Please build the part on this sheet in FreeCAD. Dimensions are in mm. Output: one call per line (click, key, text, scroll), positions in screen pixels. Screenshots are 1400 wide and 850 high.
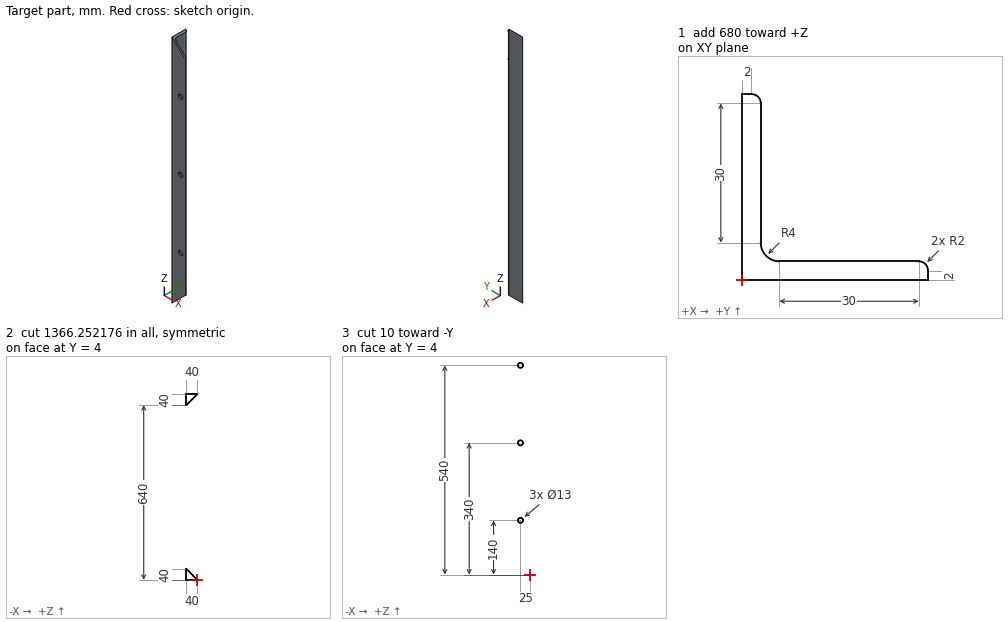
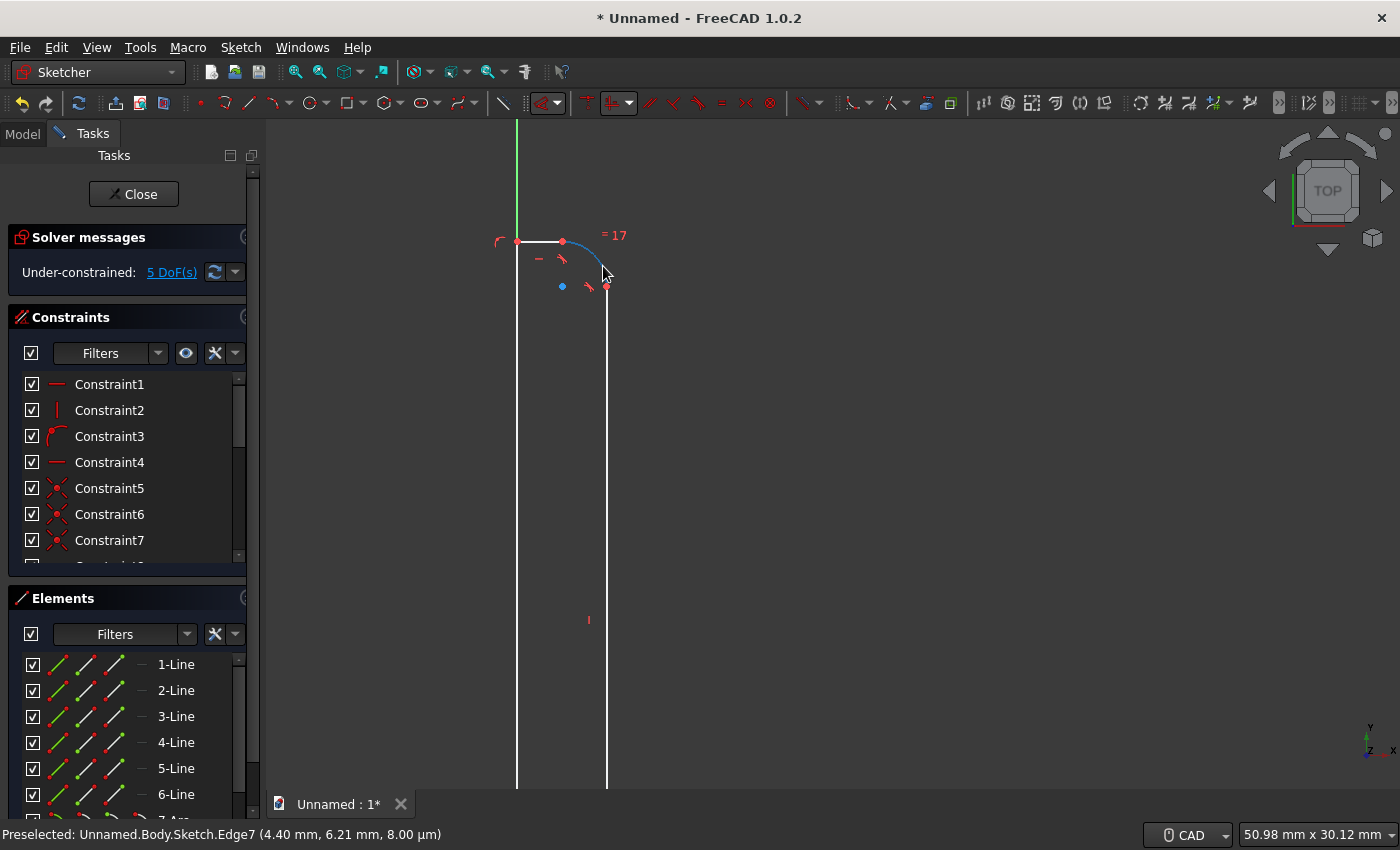
click(602, 266)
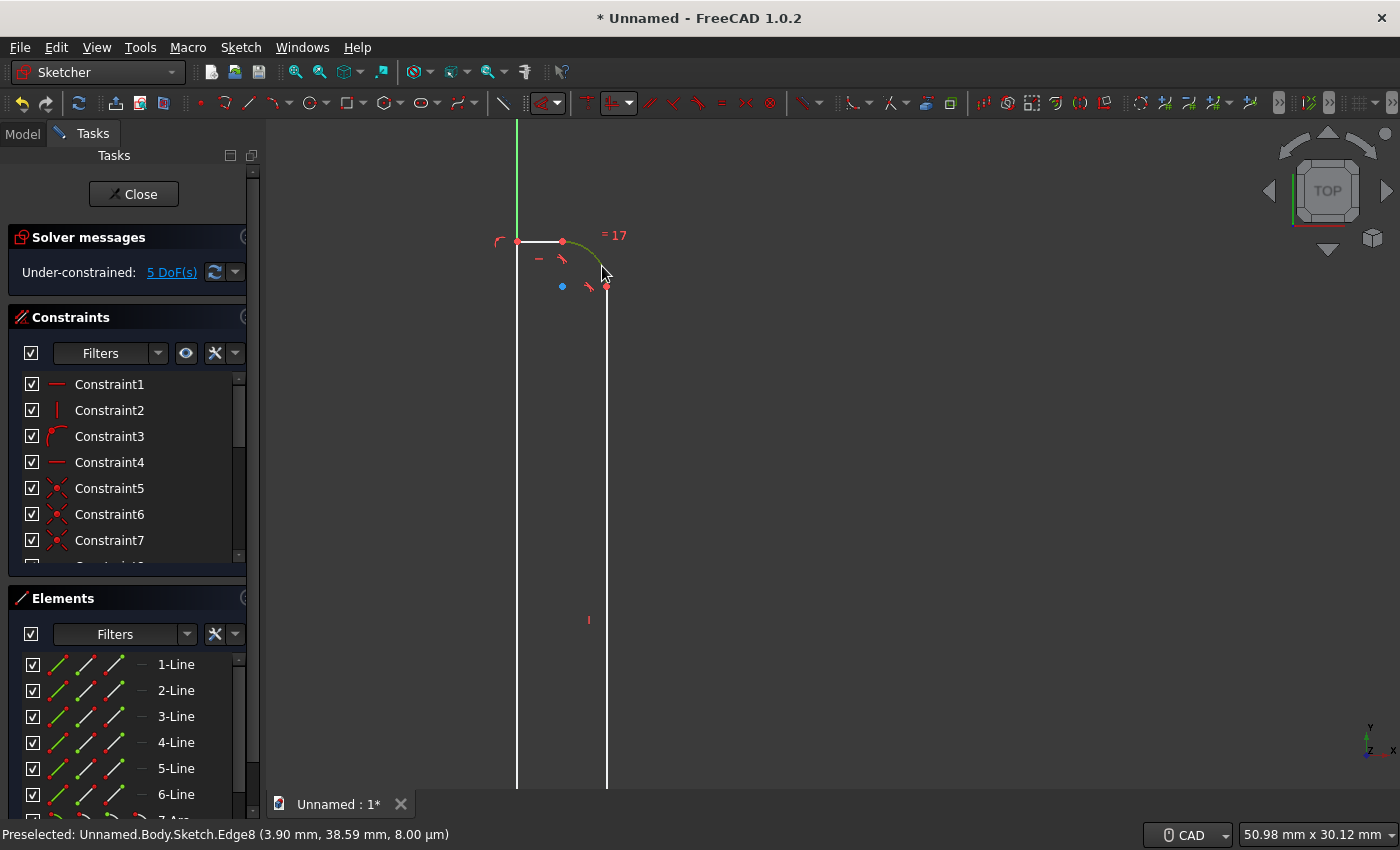
key(k)
key(r)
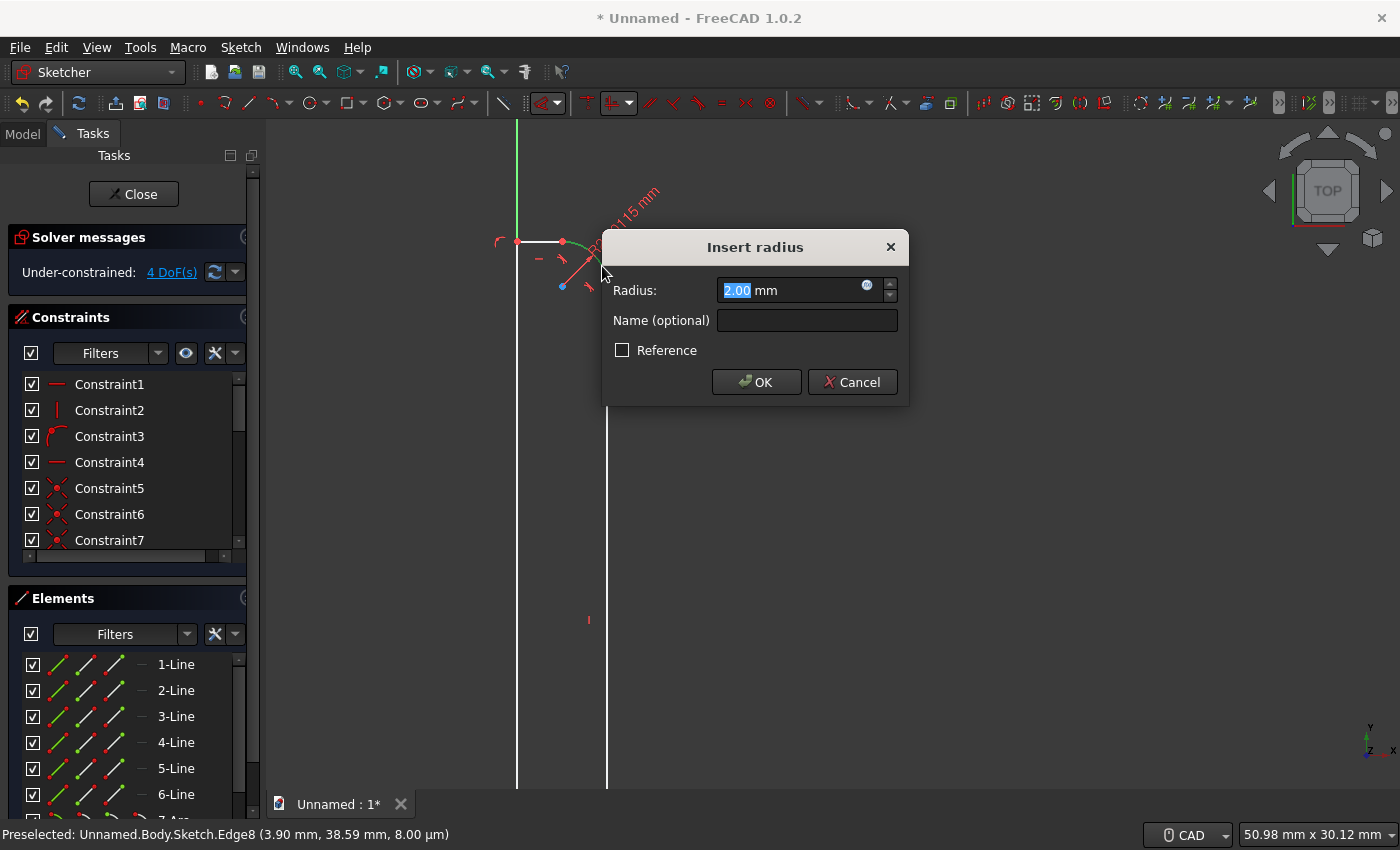
text(2)
key(Return)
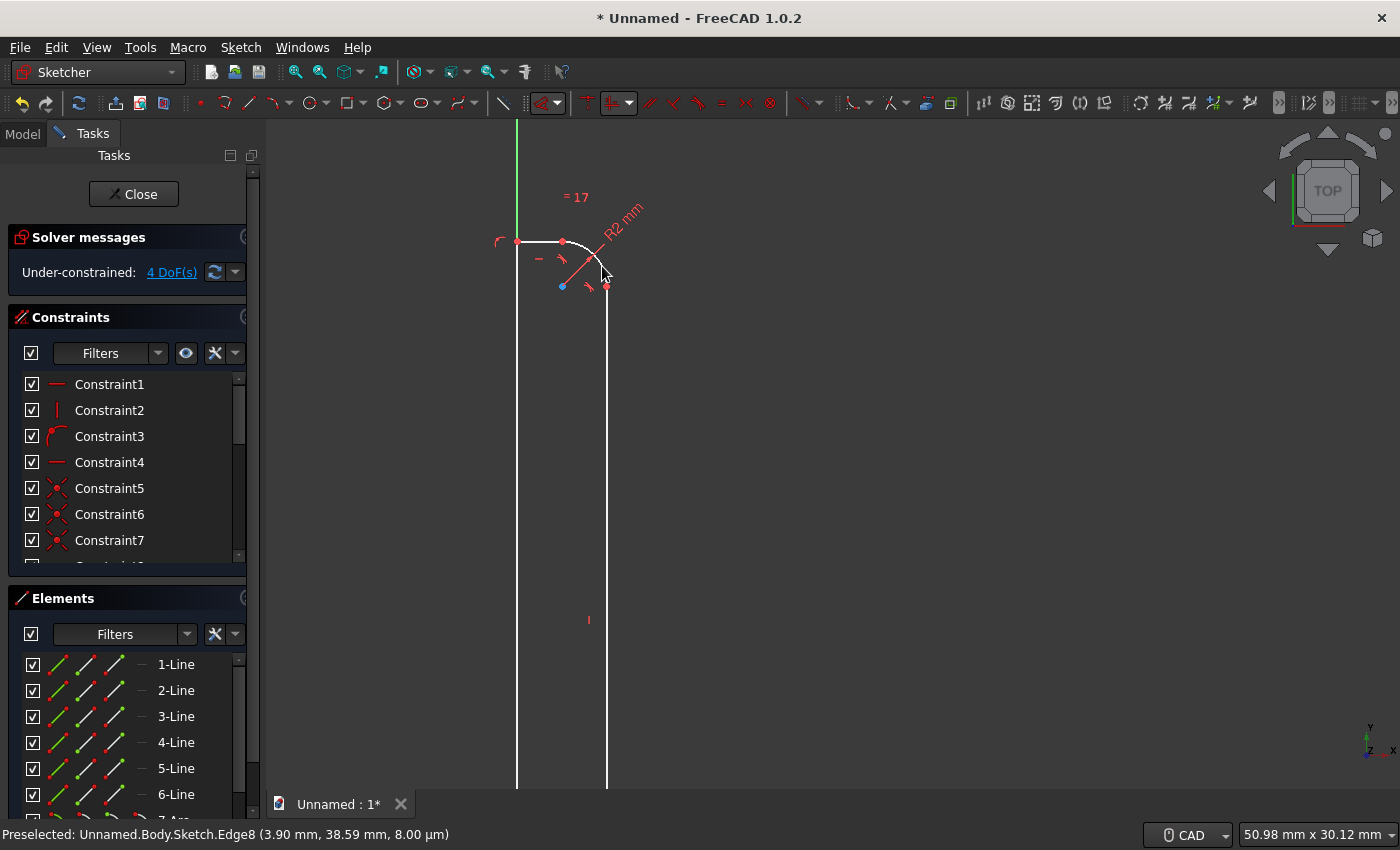
click(549, 242)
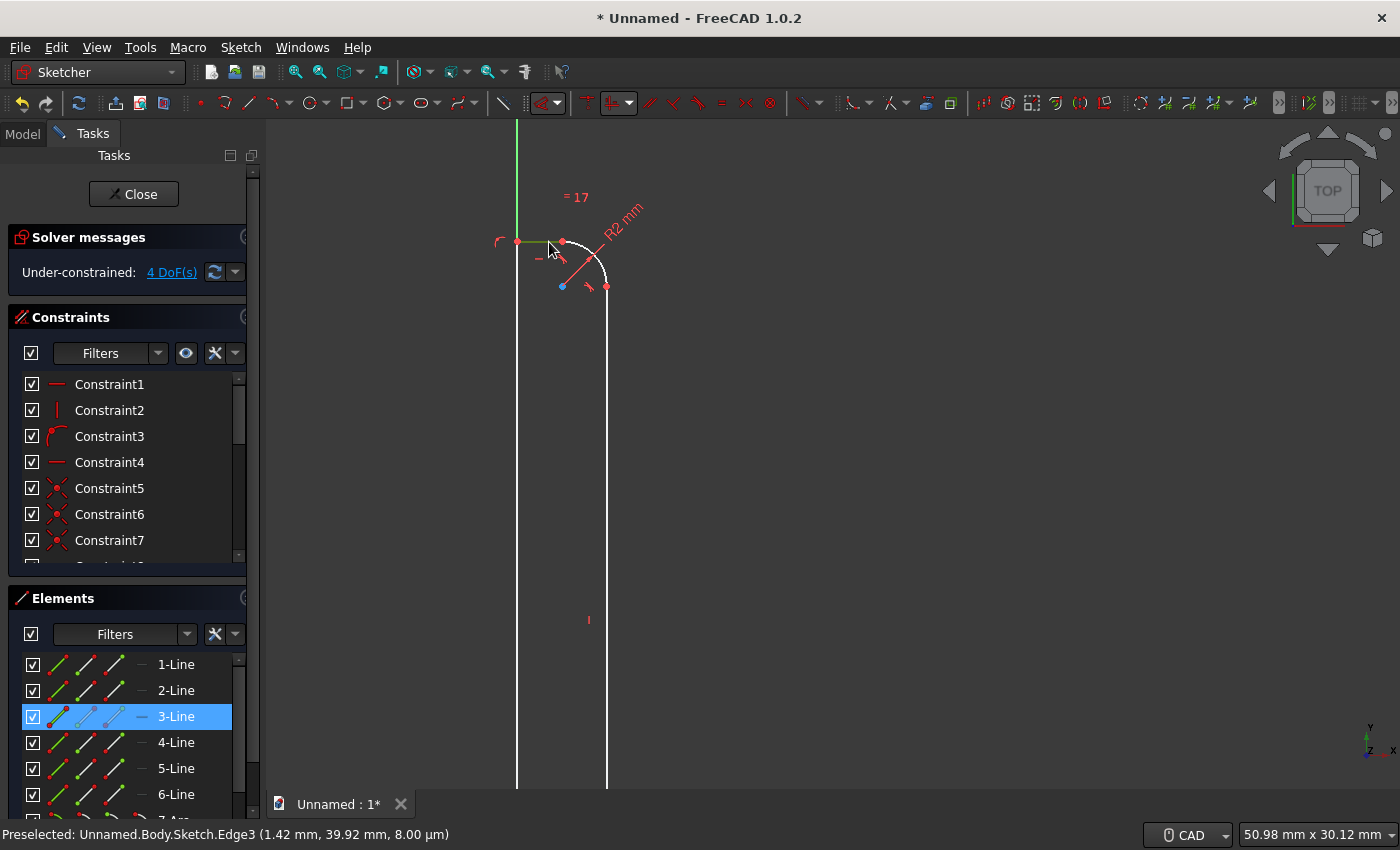
click(560, 104)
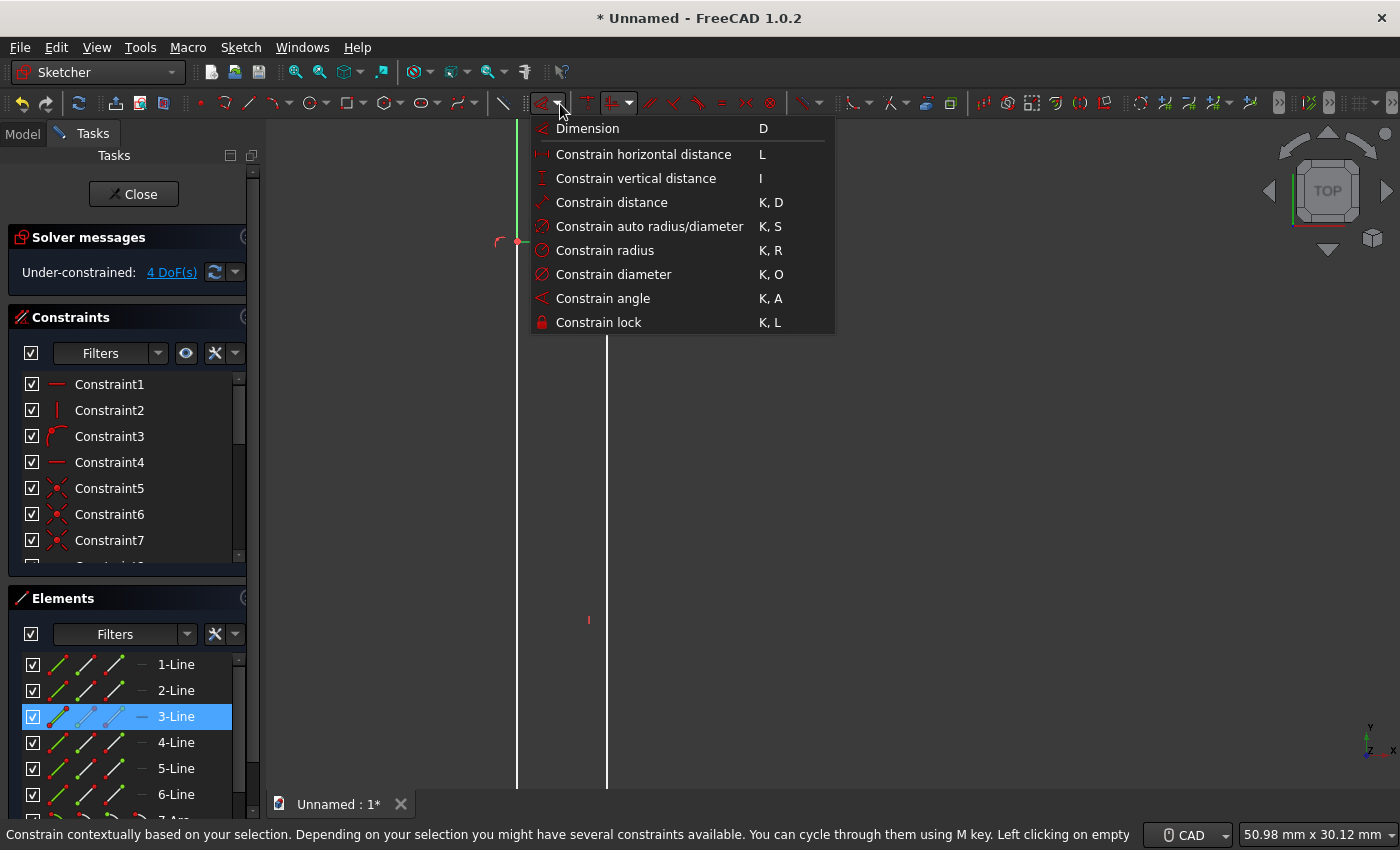
click(683, 154)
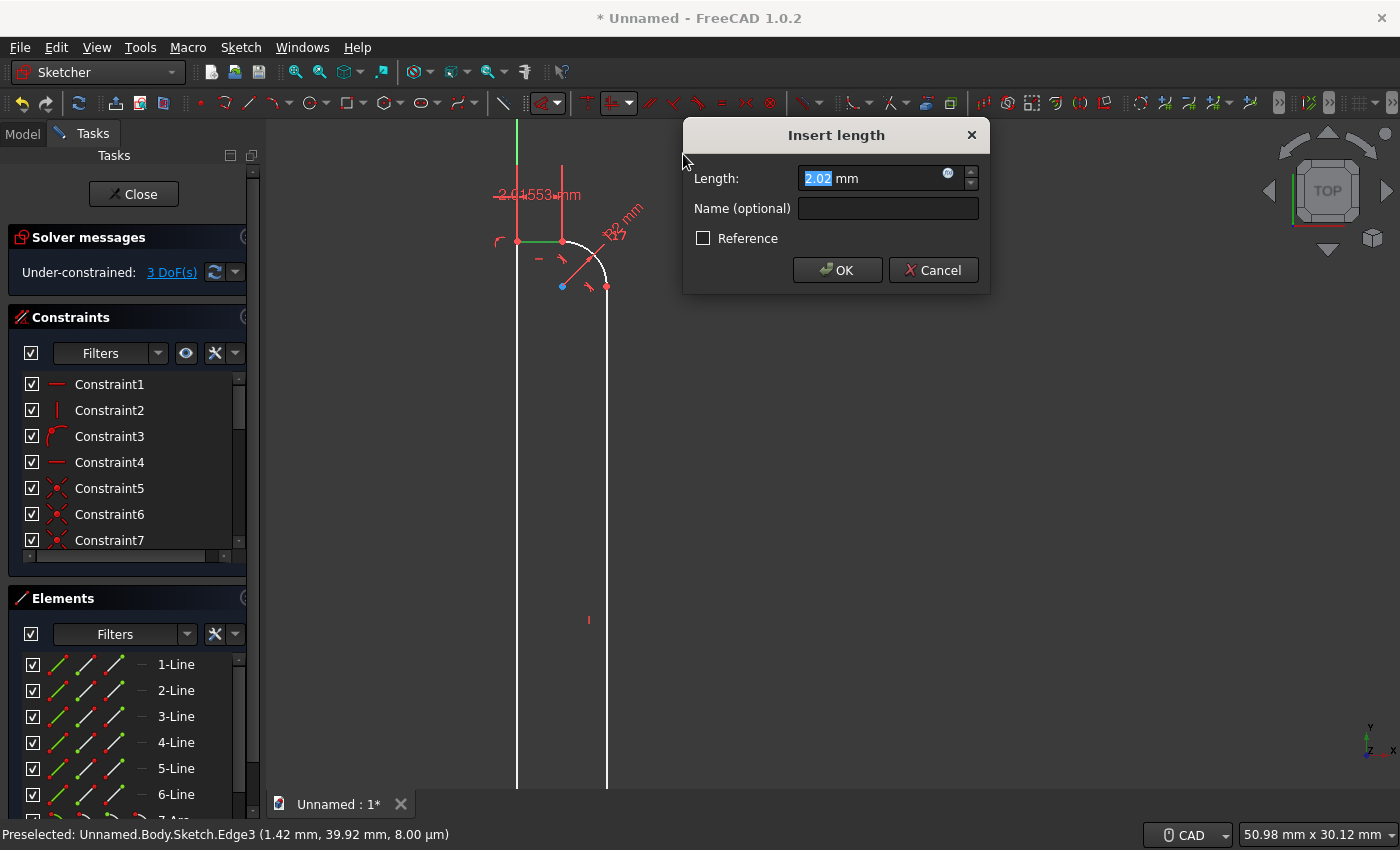
text(2)
key(Return)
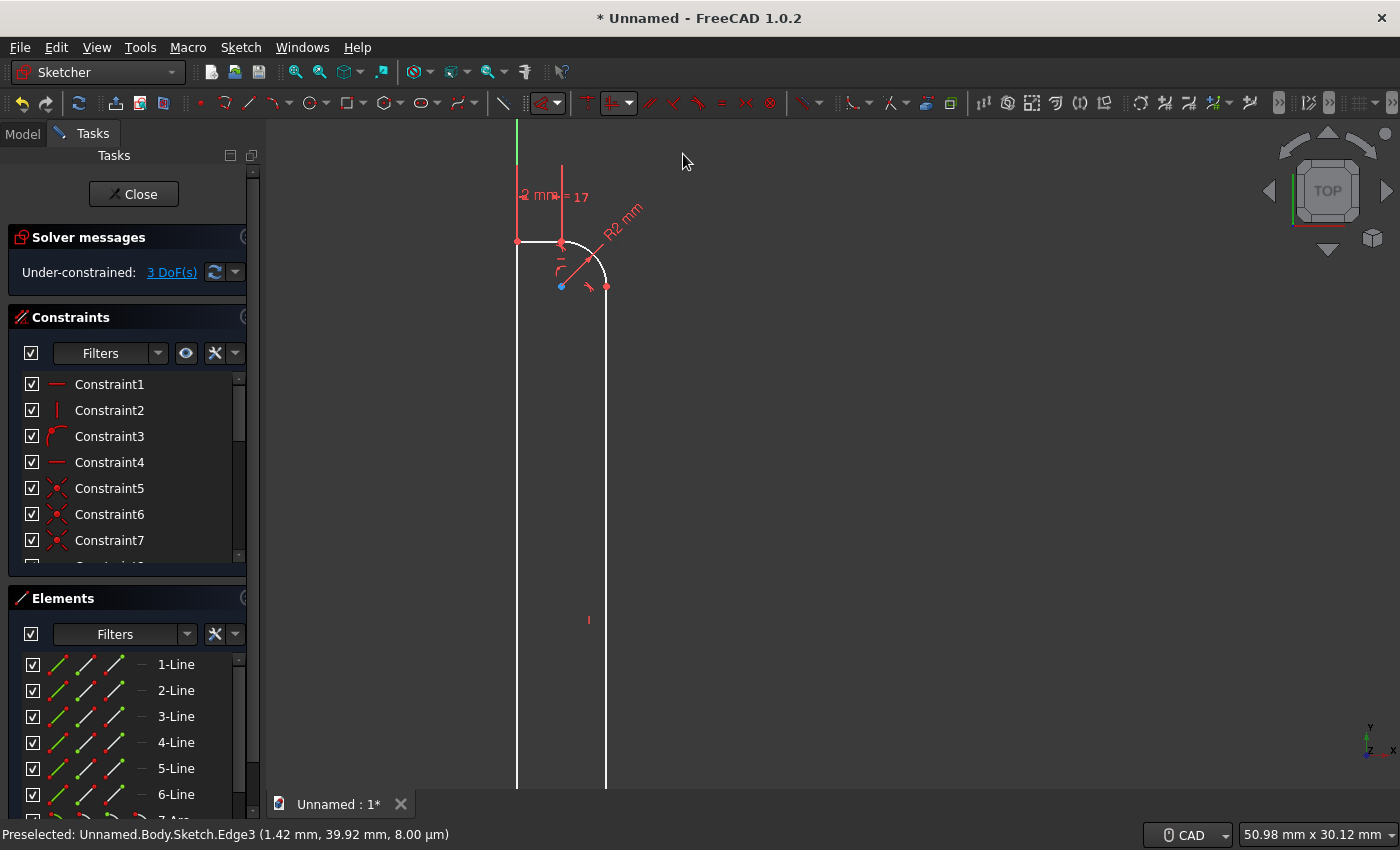
scroll(603, 266, down, 4)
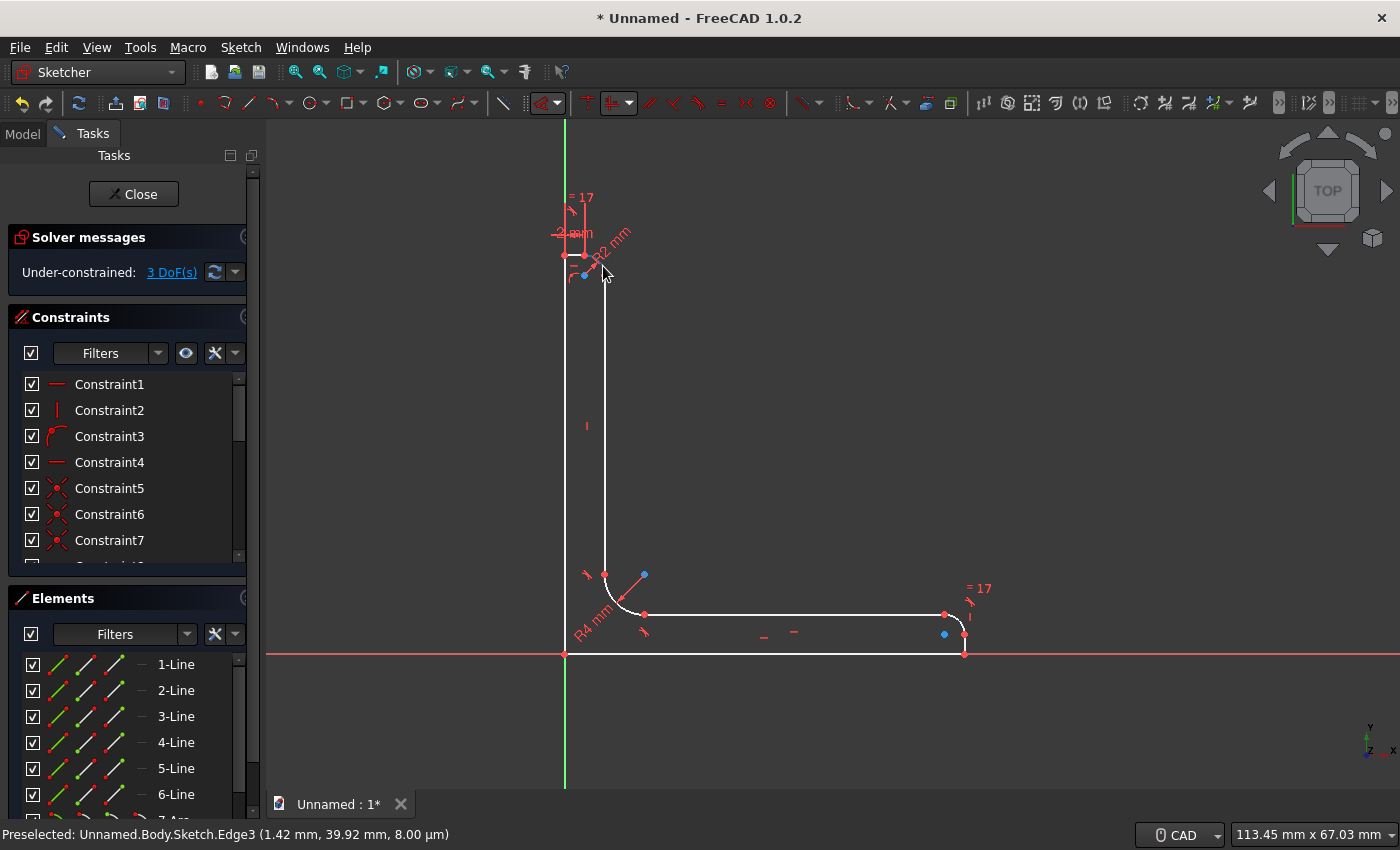
scroll(965, 648, up, 5)